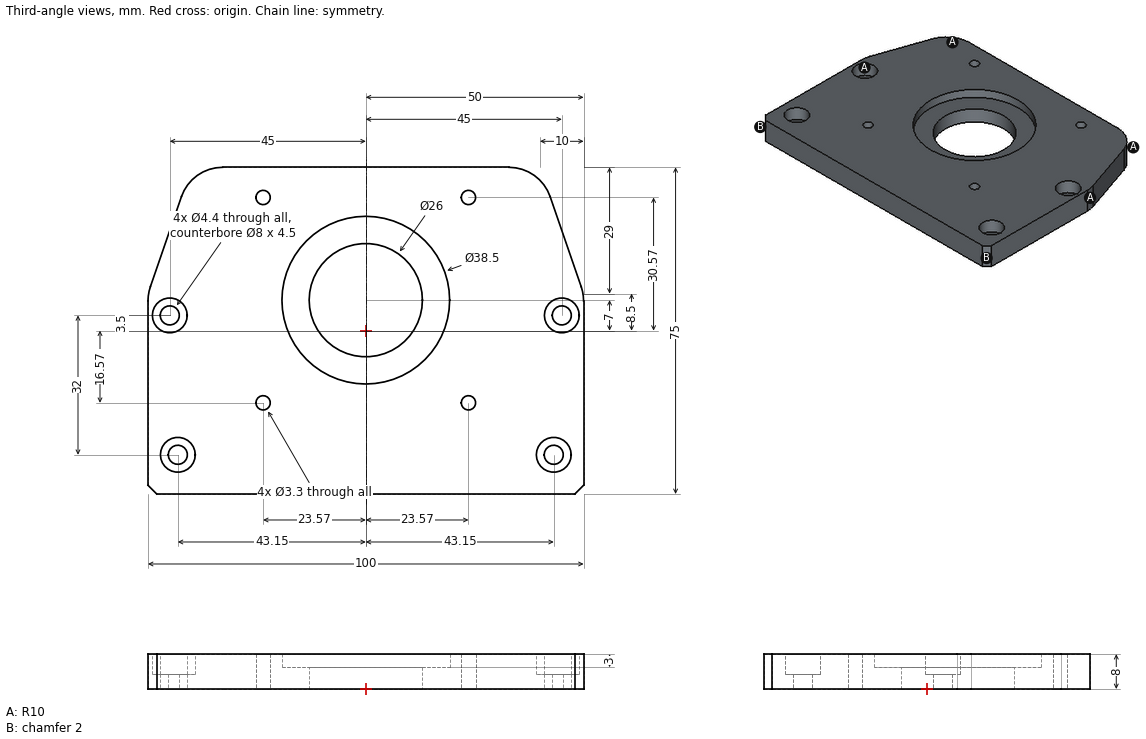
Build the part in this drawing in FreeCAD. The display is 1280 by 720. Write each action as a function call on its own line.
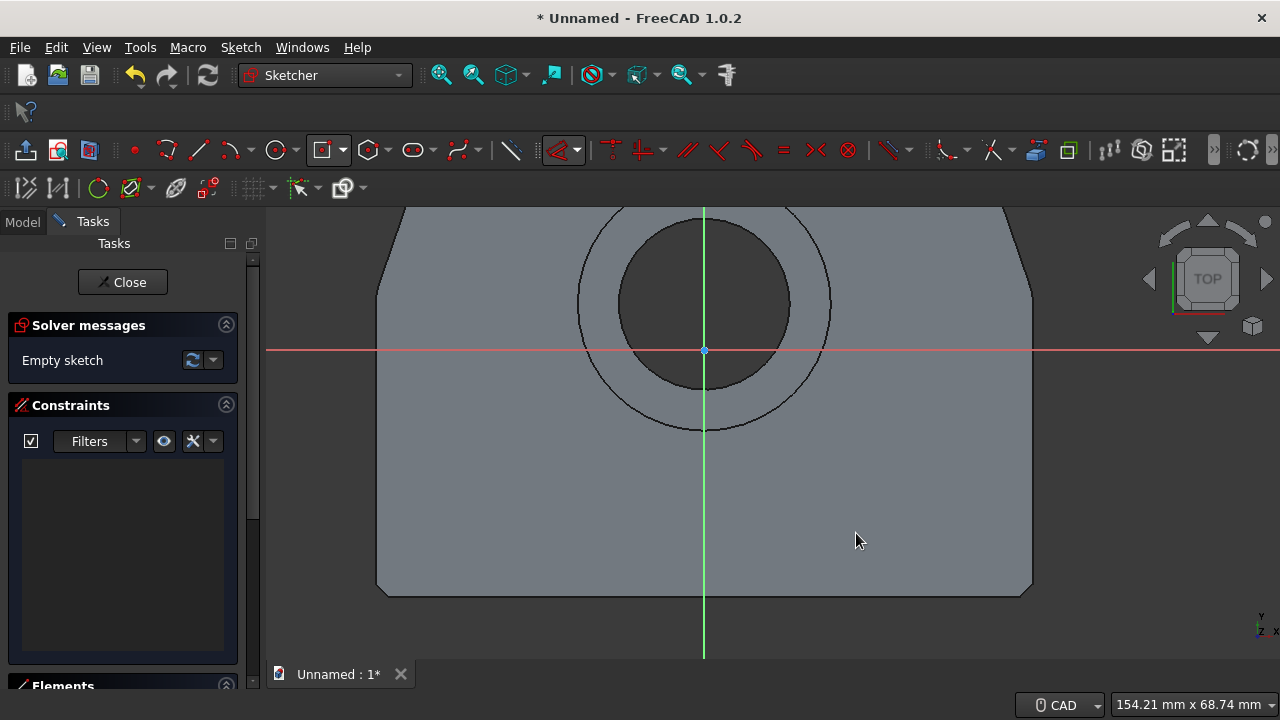
click(276, 150)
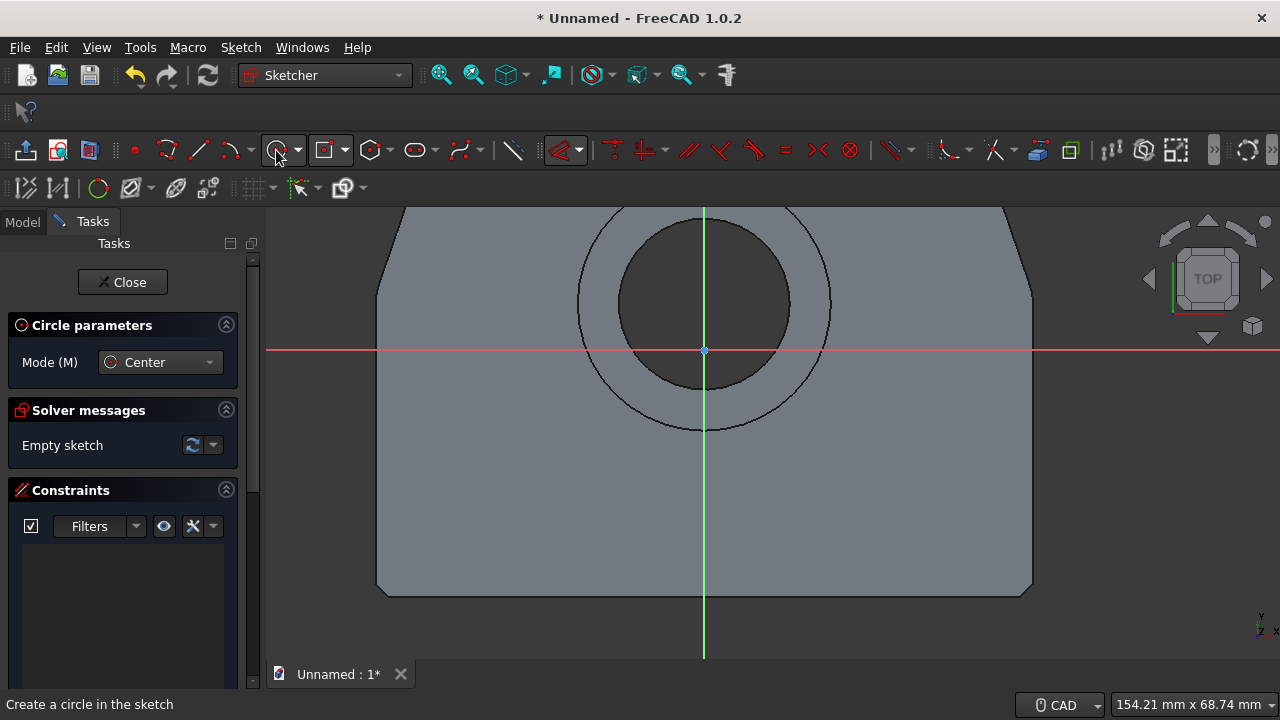
scroll(408, 327, up, 3)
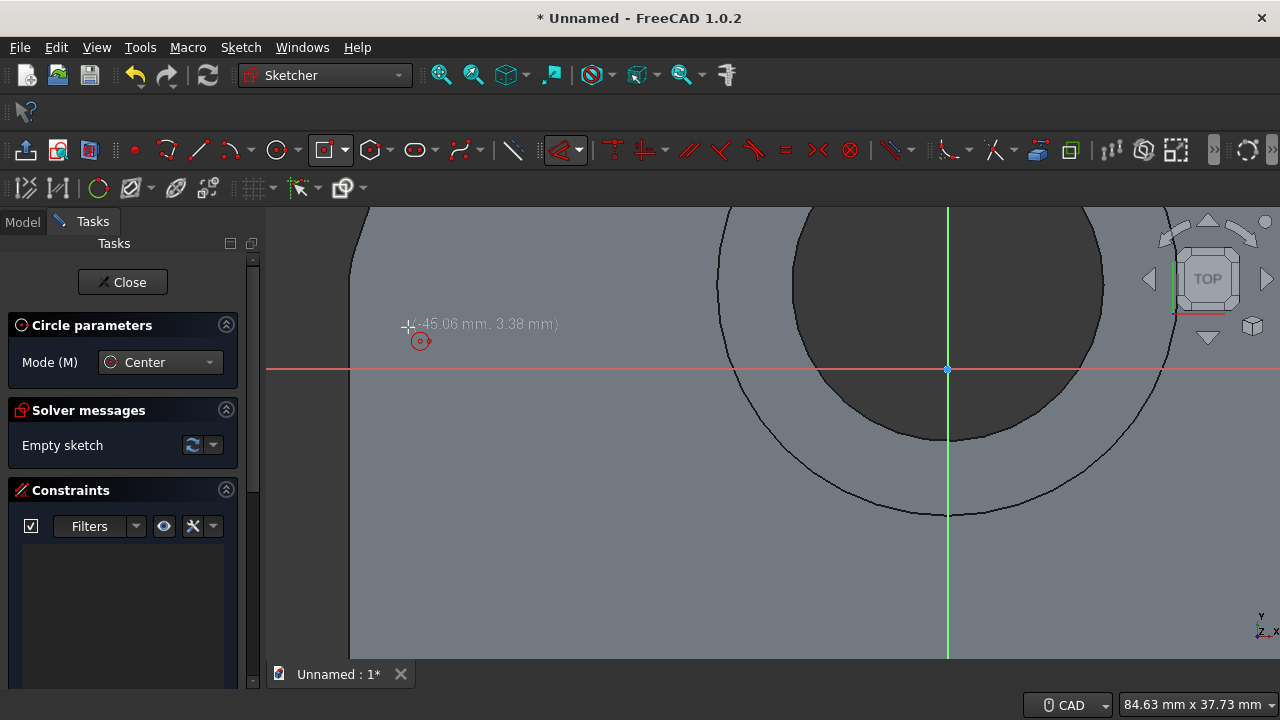
click(409, 327)
click(427, 308)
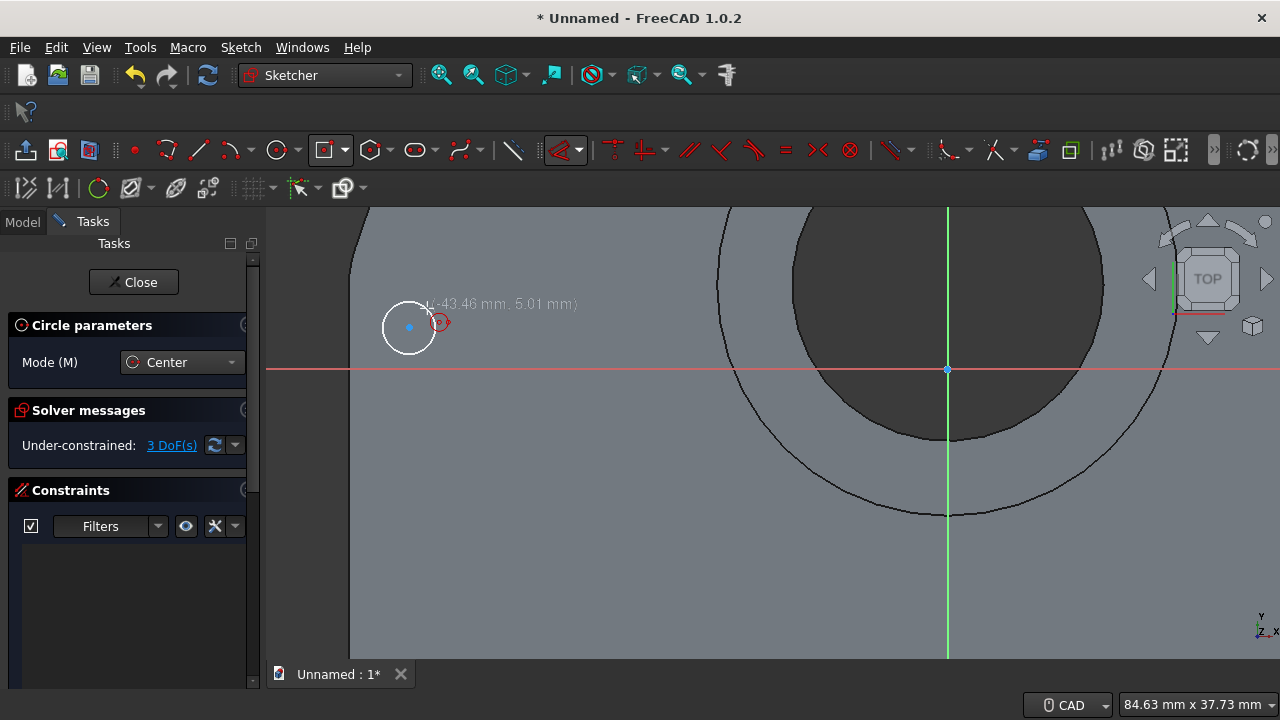
scroll(409, 329, down, 3)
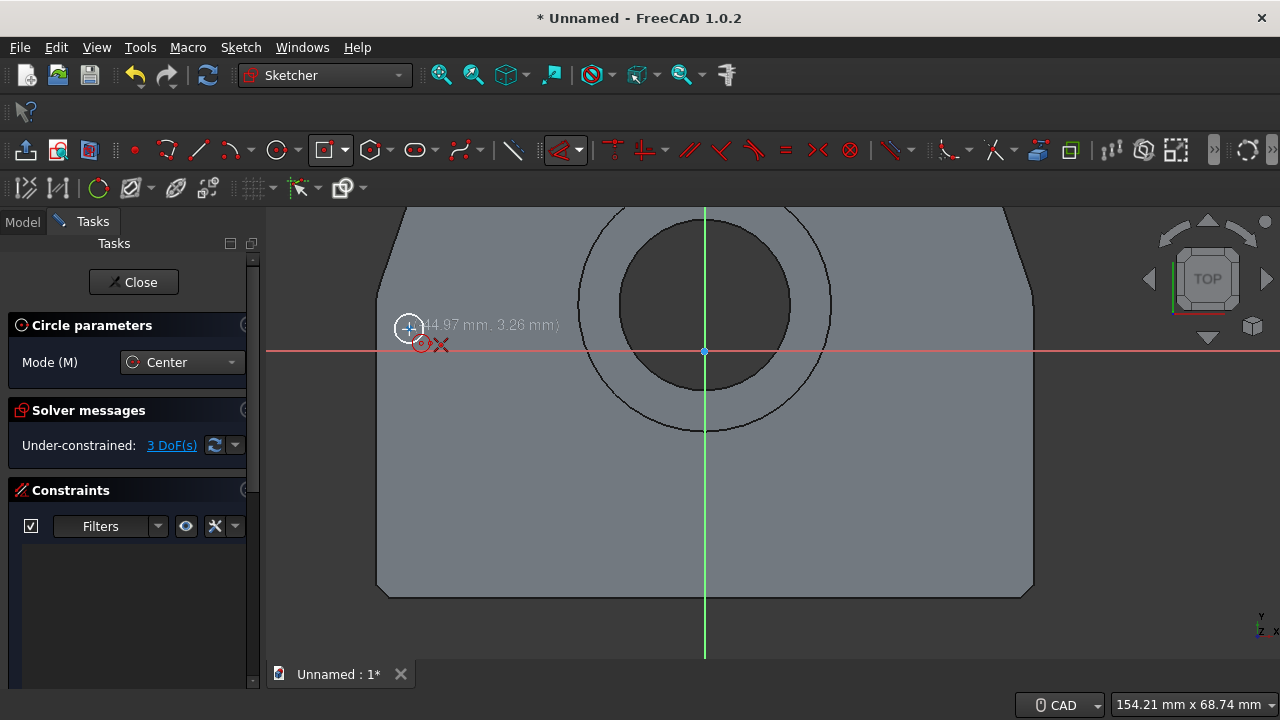
scroll(421, 538, up, 3)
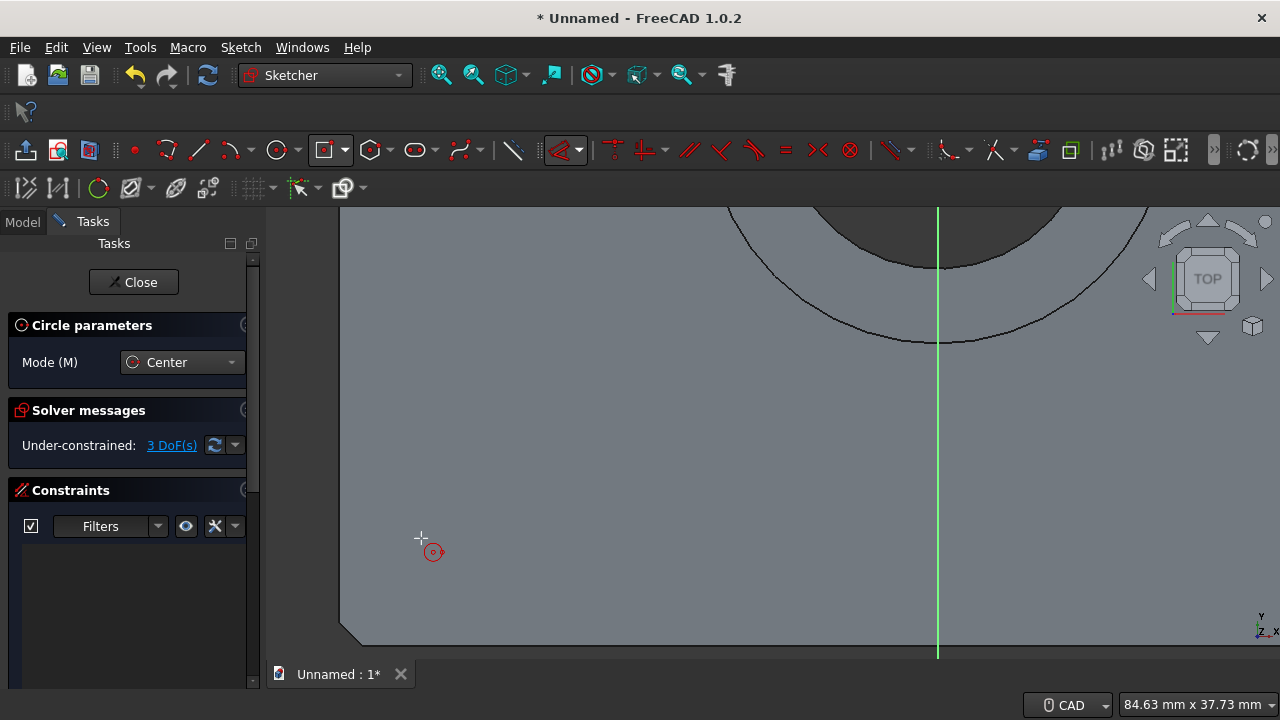
click(421, 538)
click(440, 520)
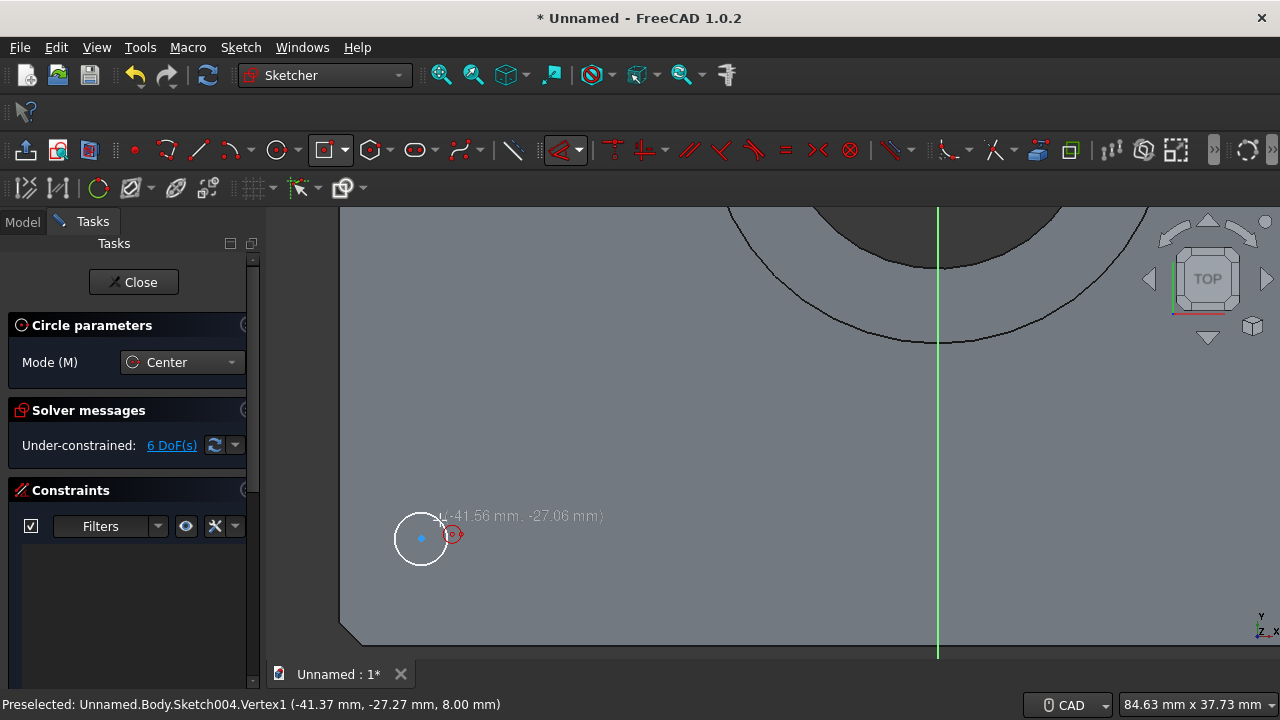
scroll(421, 538, down, 3)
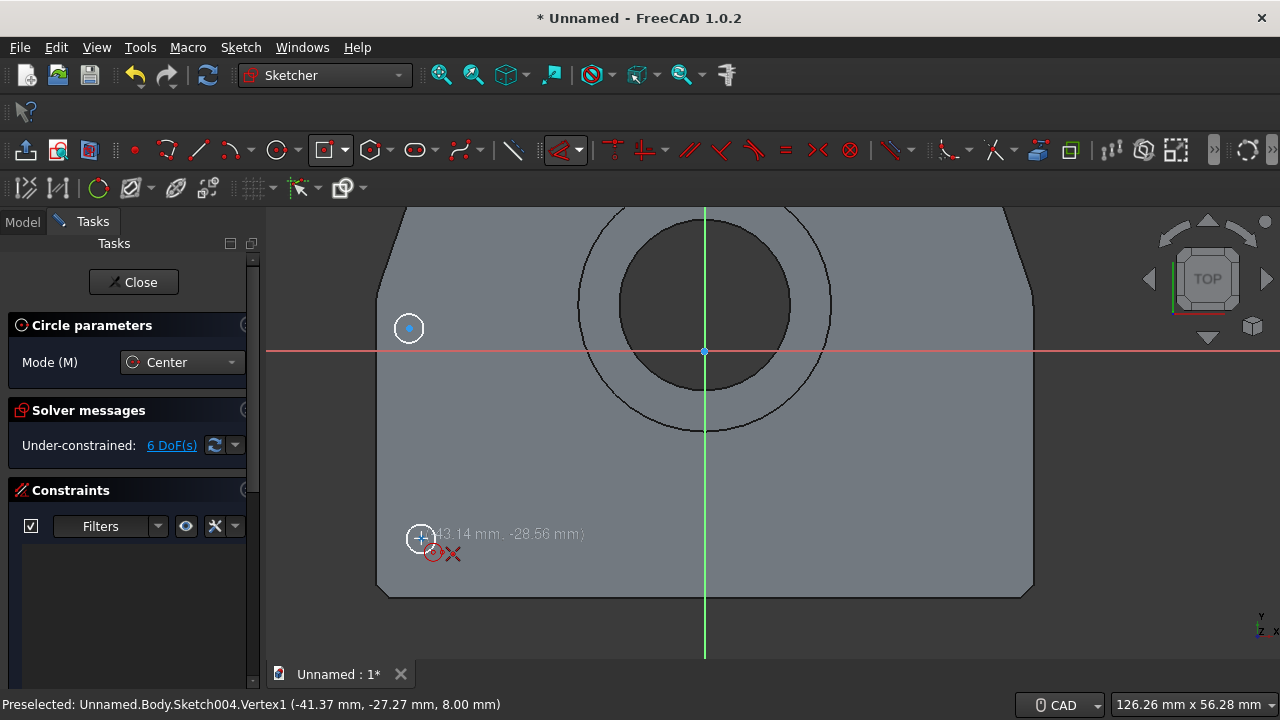
scroll(988, 538, up, 3)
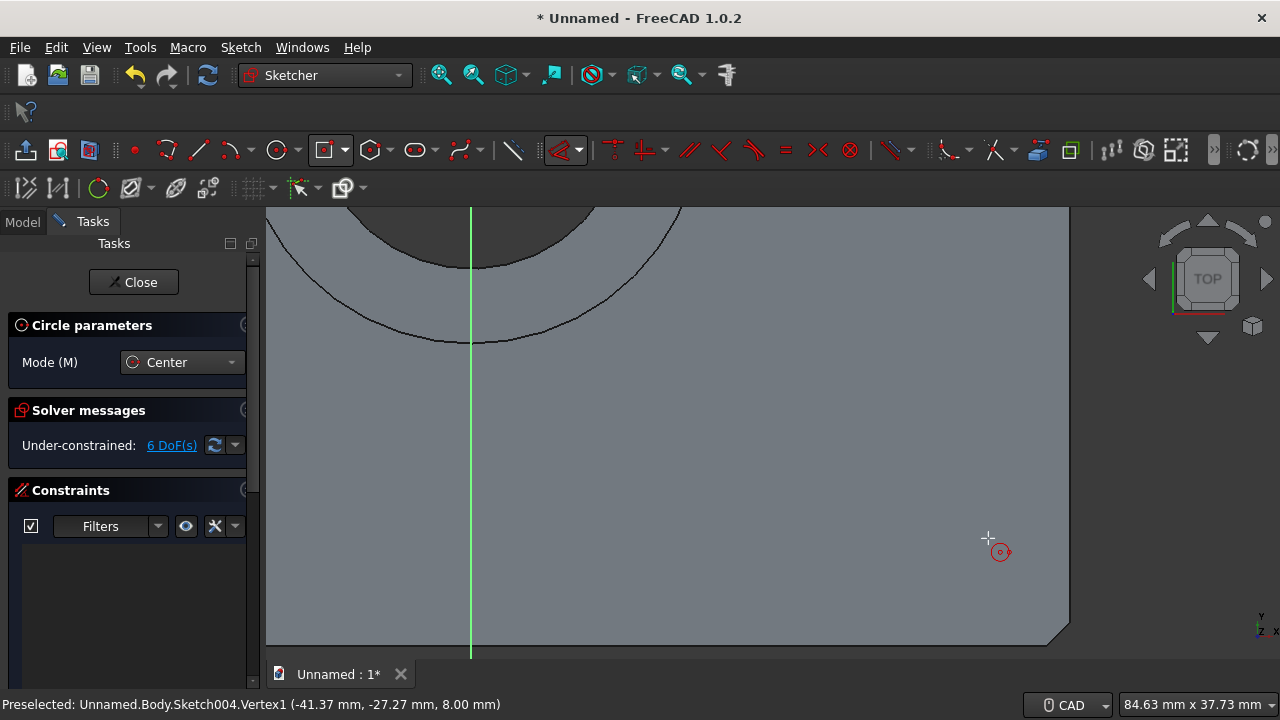
click(988, 538)
click(1007, 520)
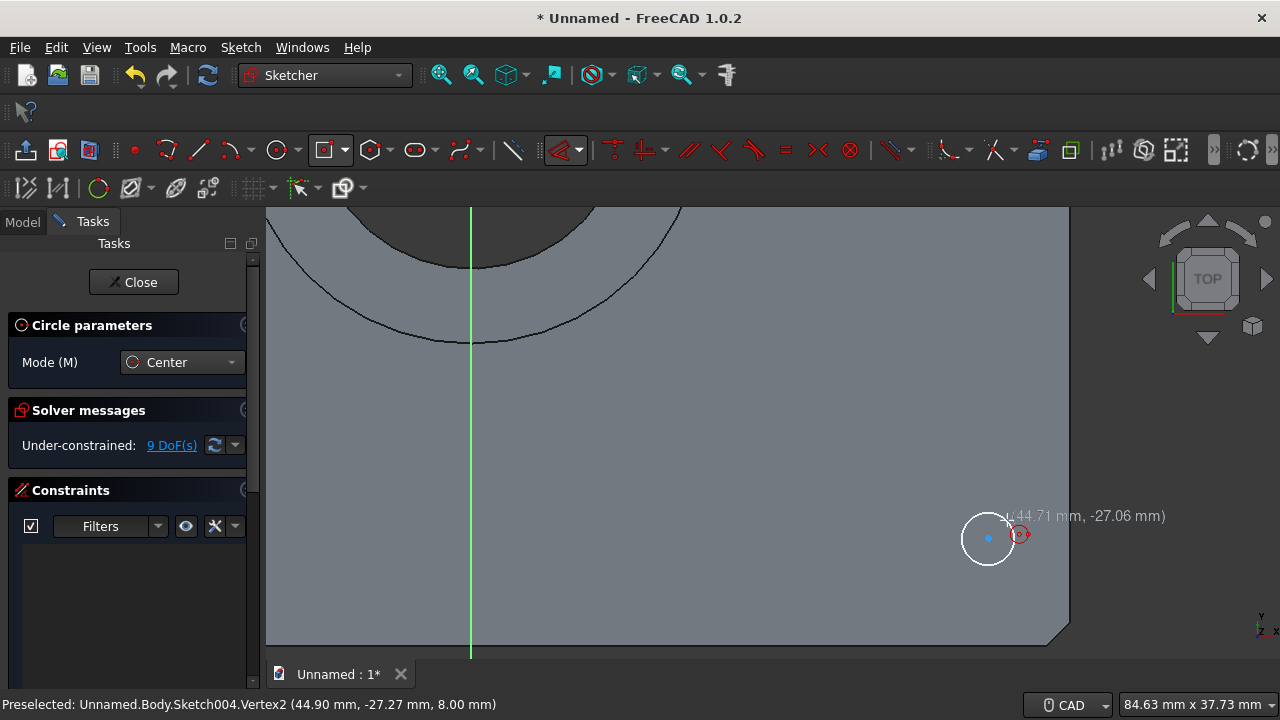
scroll(988, 538, down, 3)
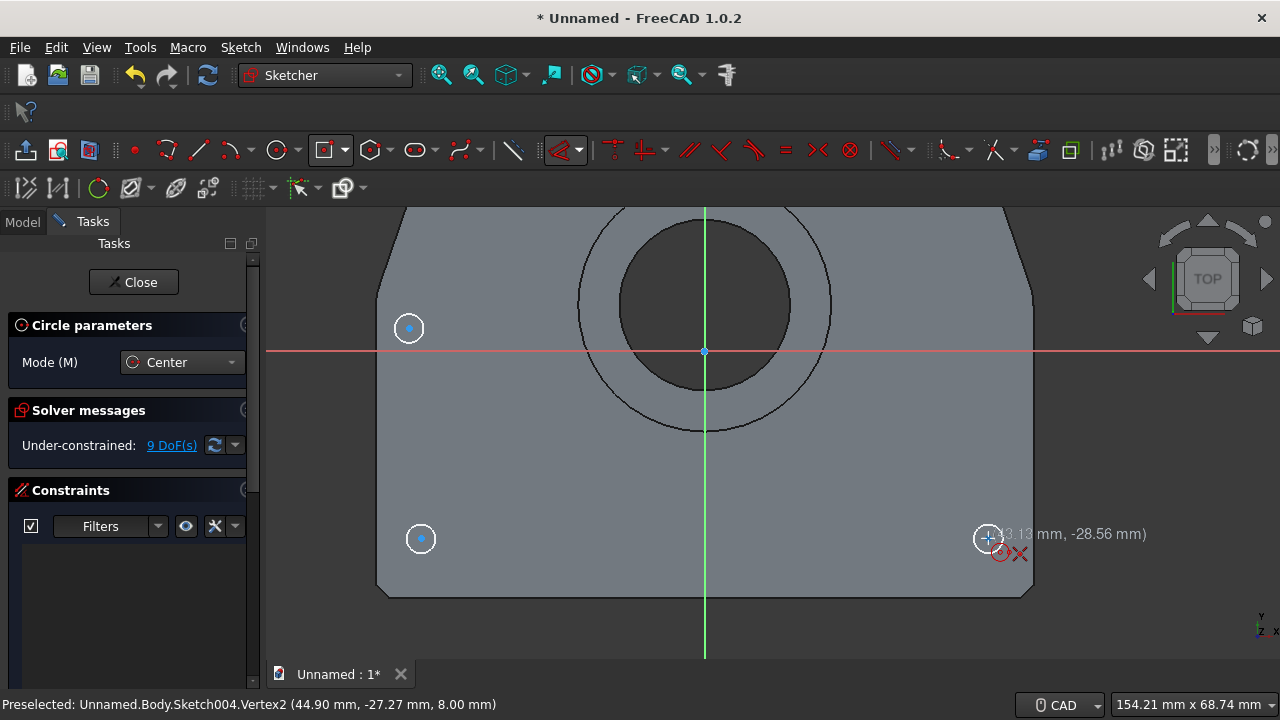
scroll(1001, 328, up, 3)